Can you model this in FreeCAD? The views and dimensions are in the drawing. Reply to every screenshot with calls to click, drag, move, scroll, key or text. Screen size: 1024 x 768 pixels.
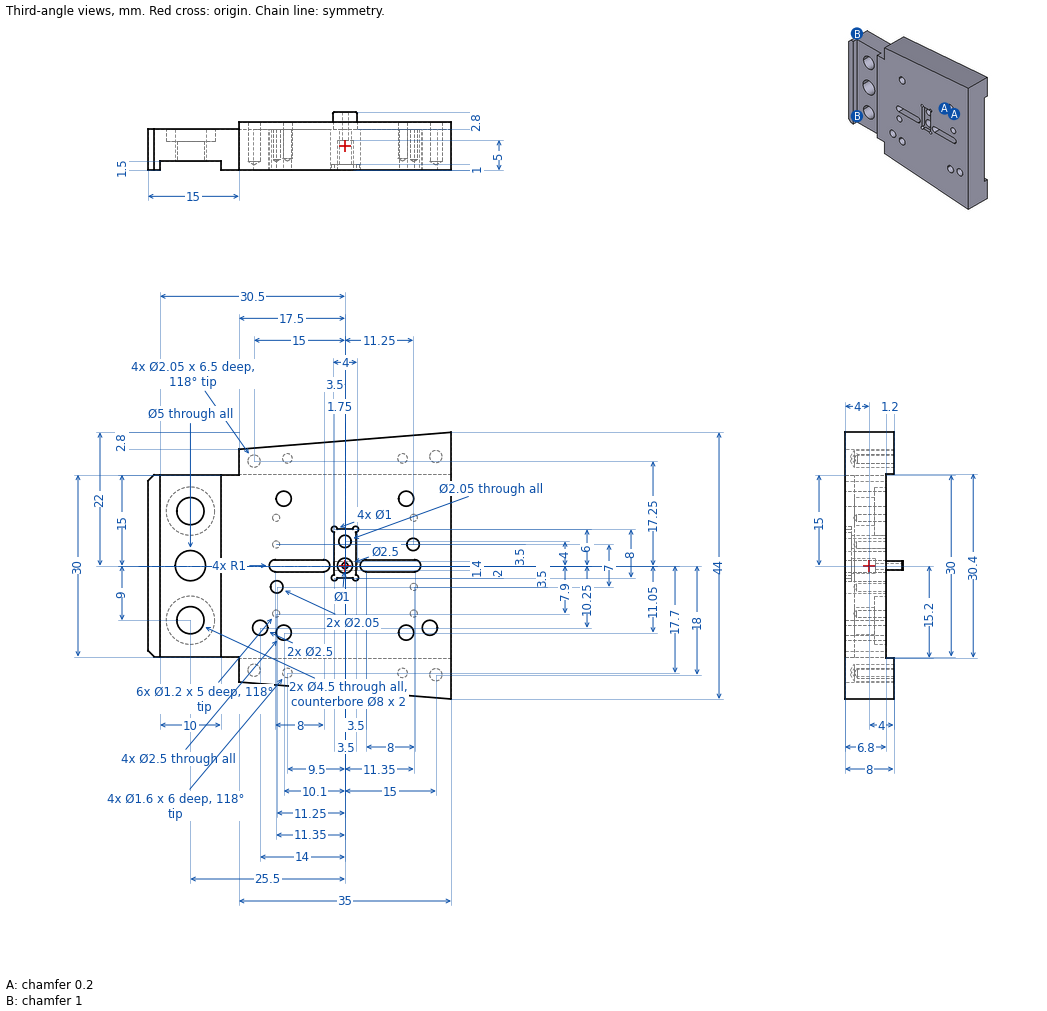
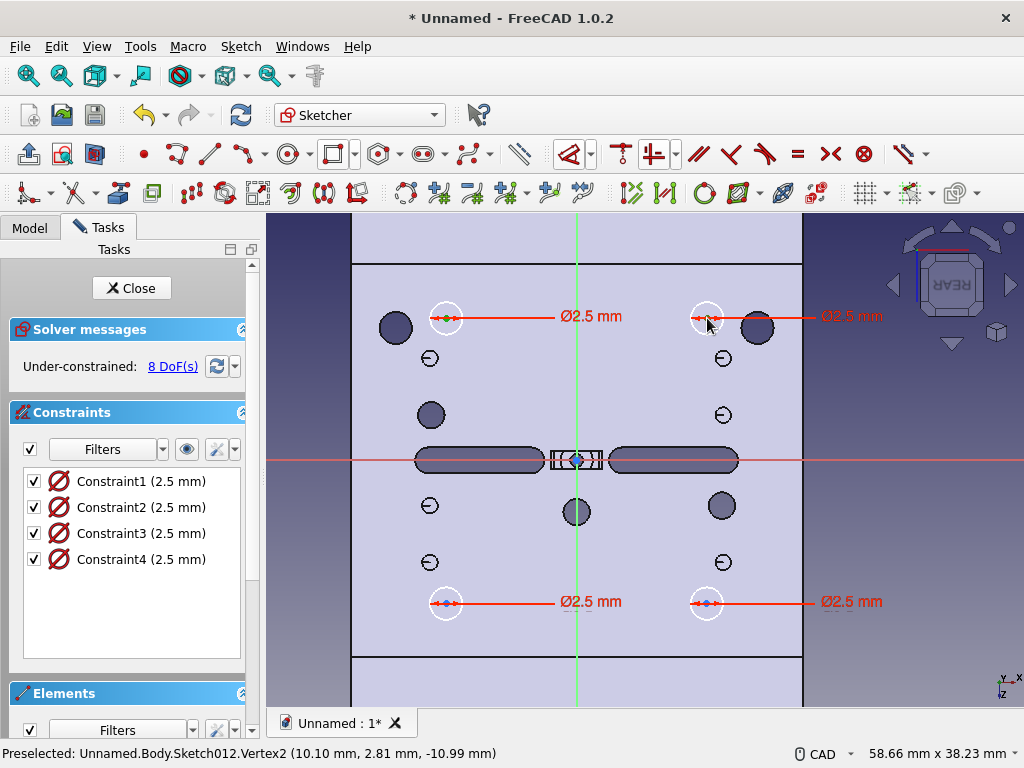
click(577, 648)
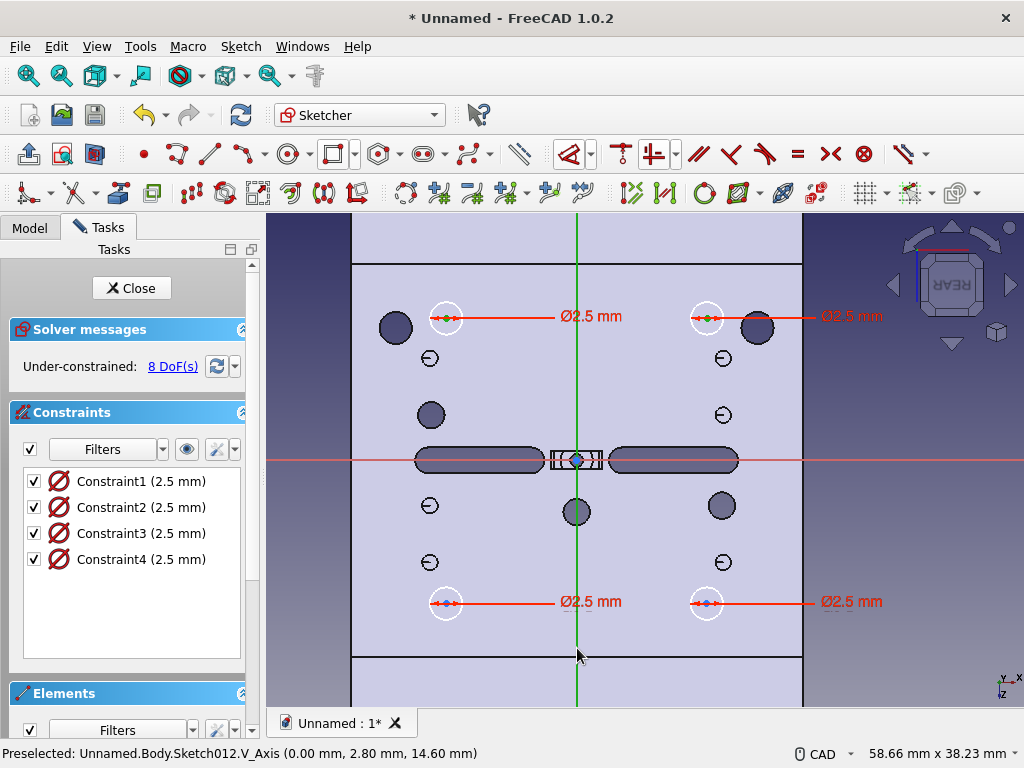
click(831, 154)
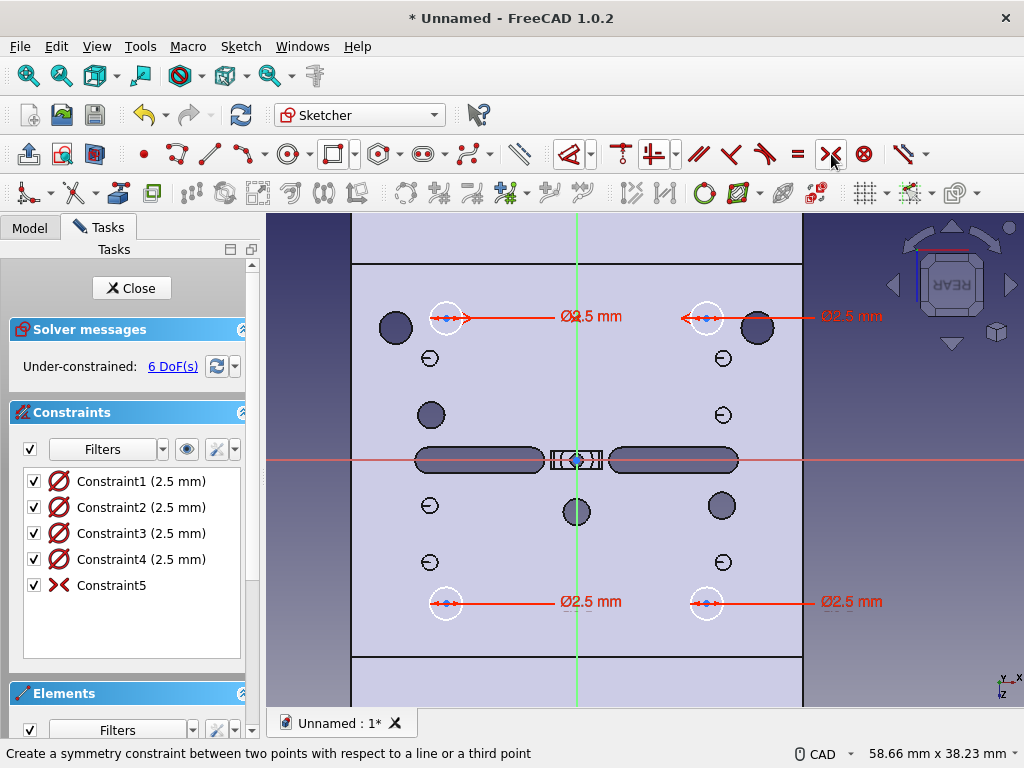
click(446, 318)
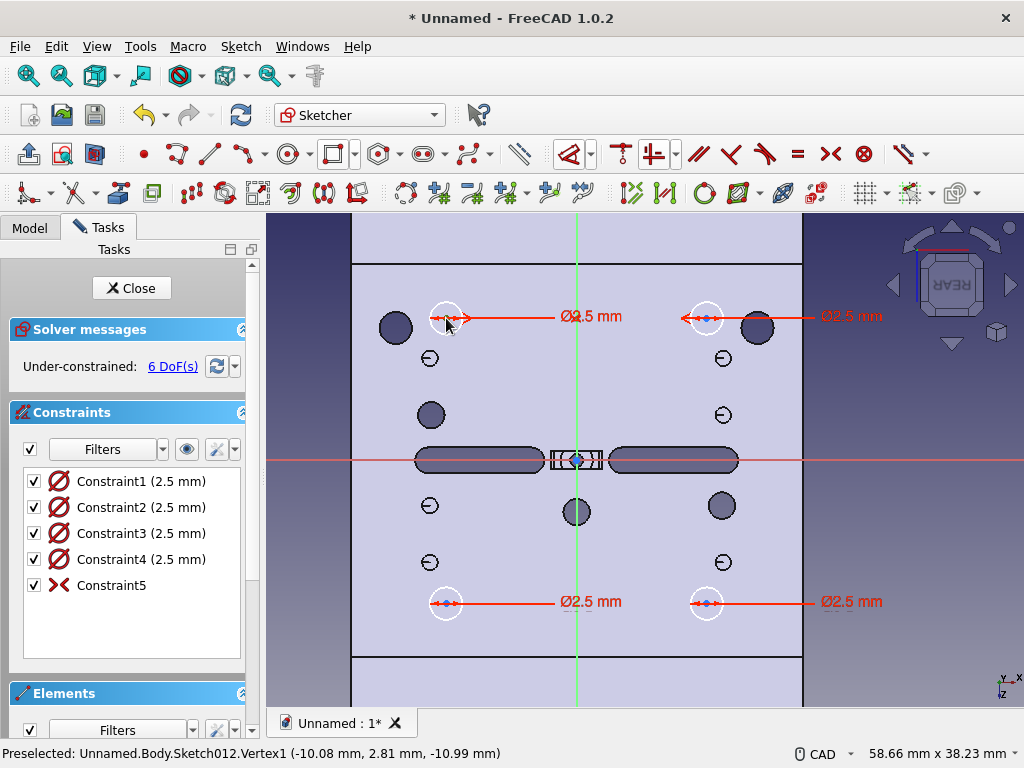
click(446, 604)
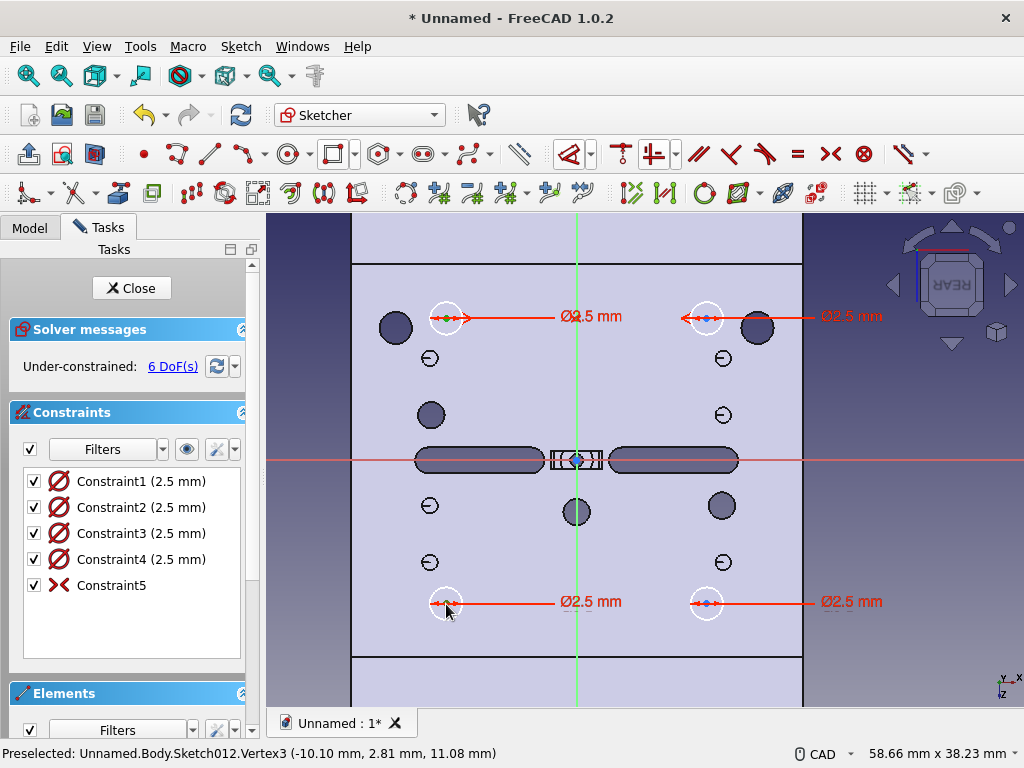
click(334, 460)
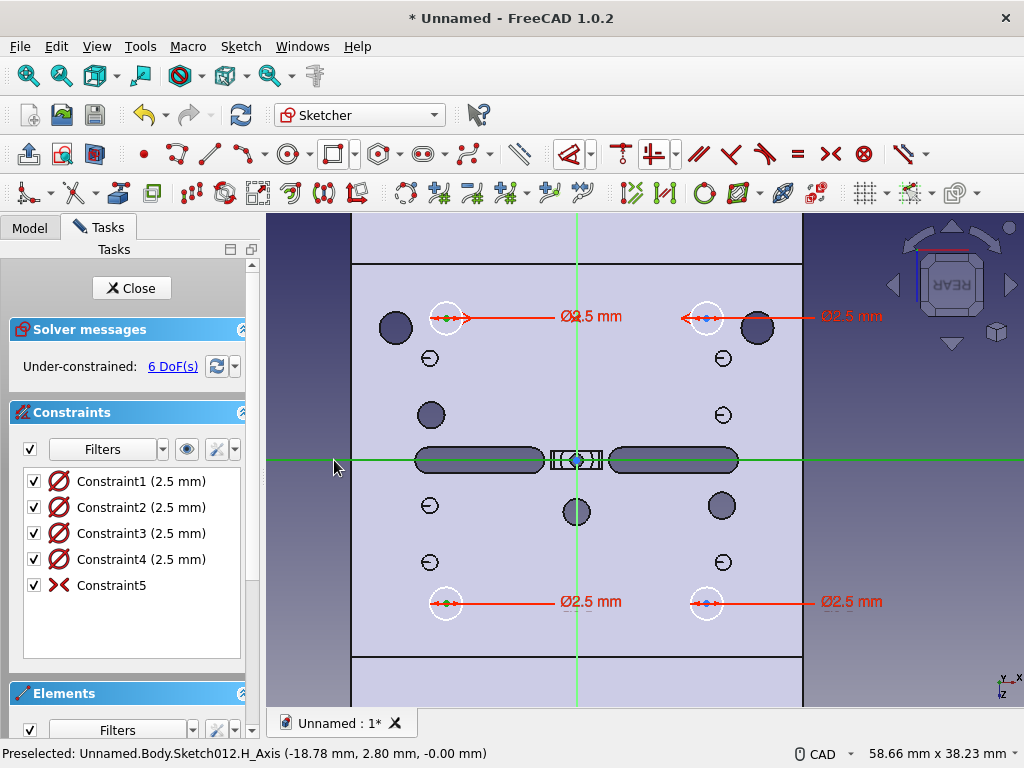
click(831, 154)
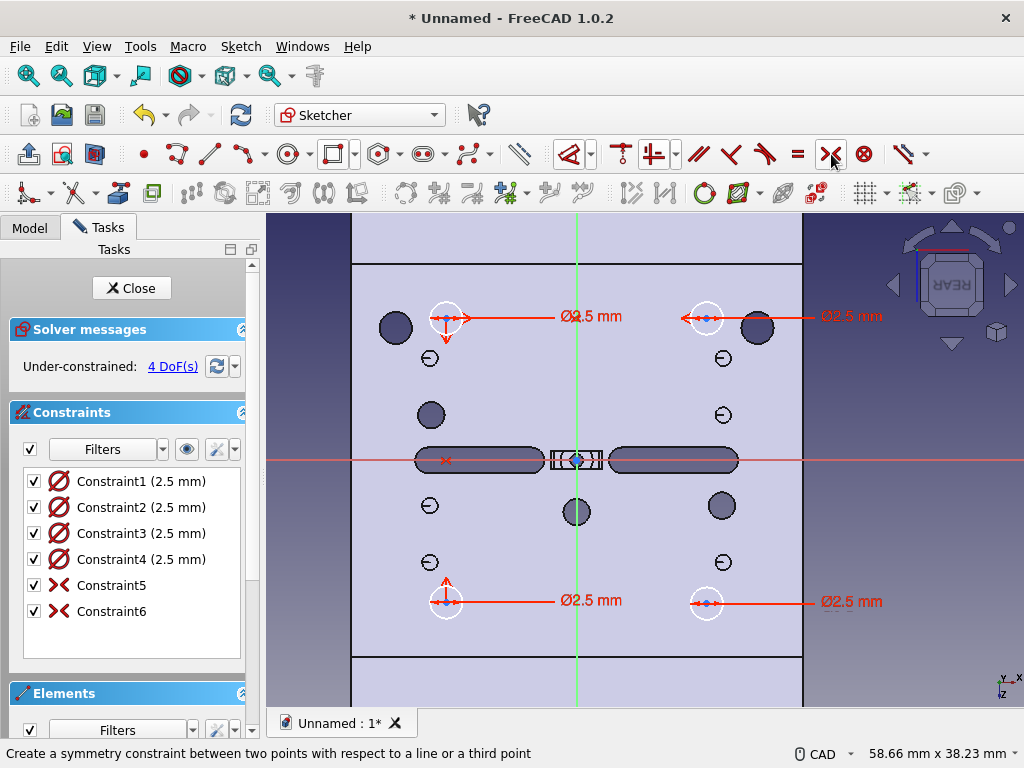
click(707, 318)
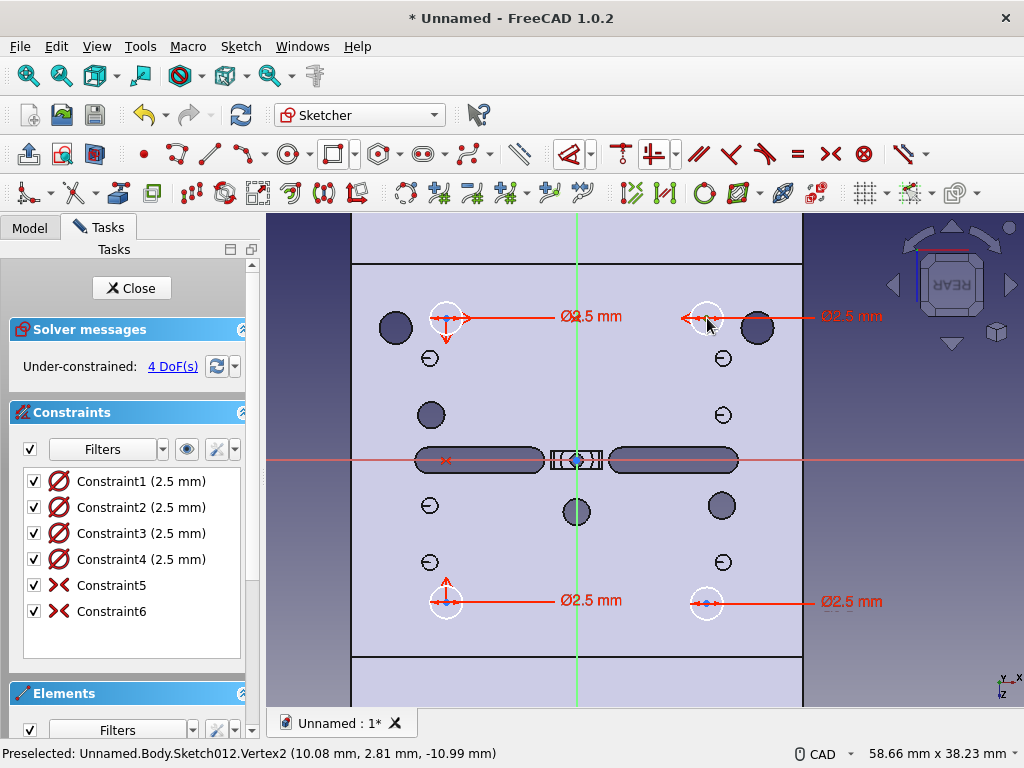
click(707, 604)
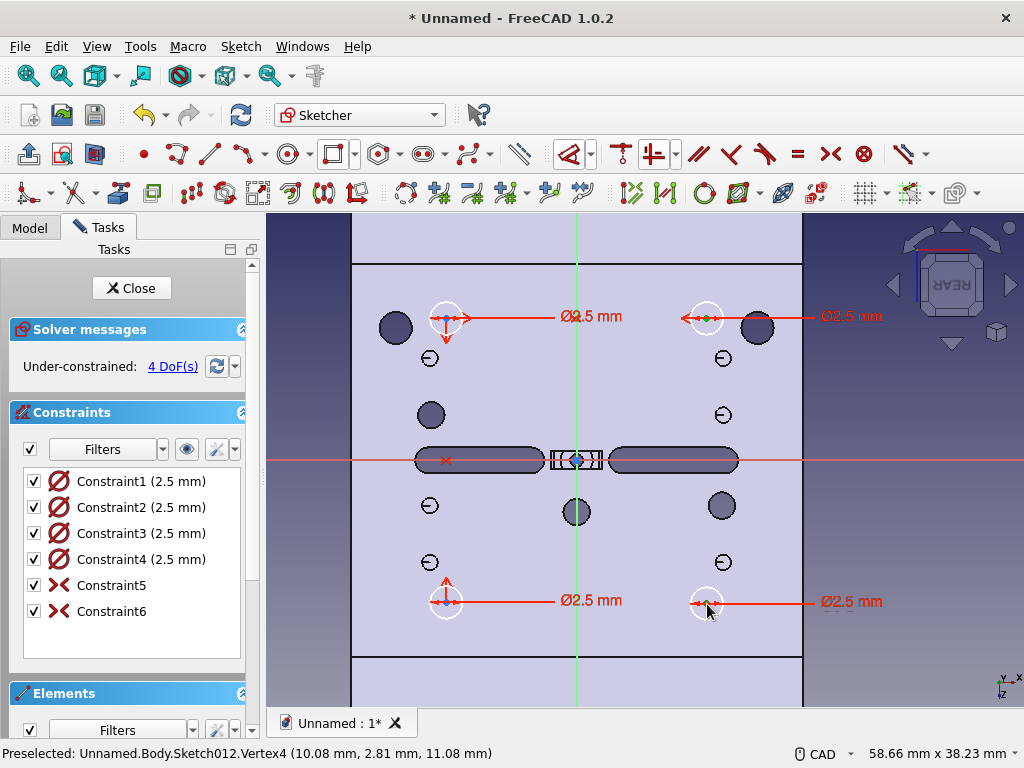
click(334, 460)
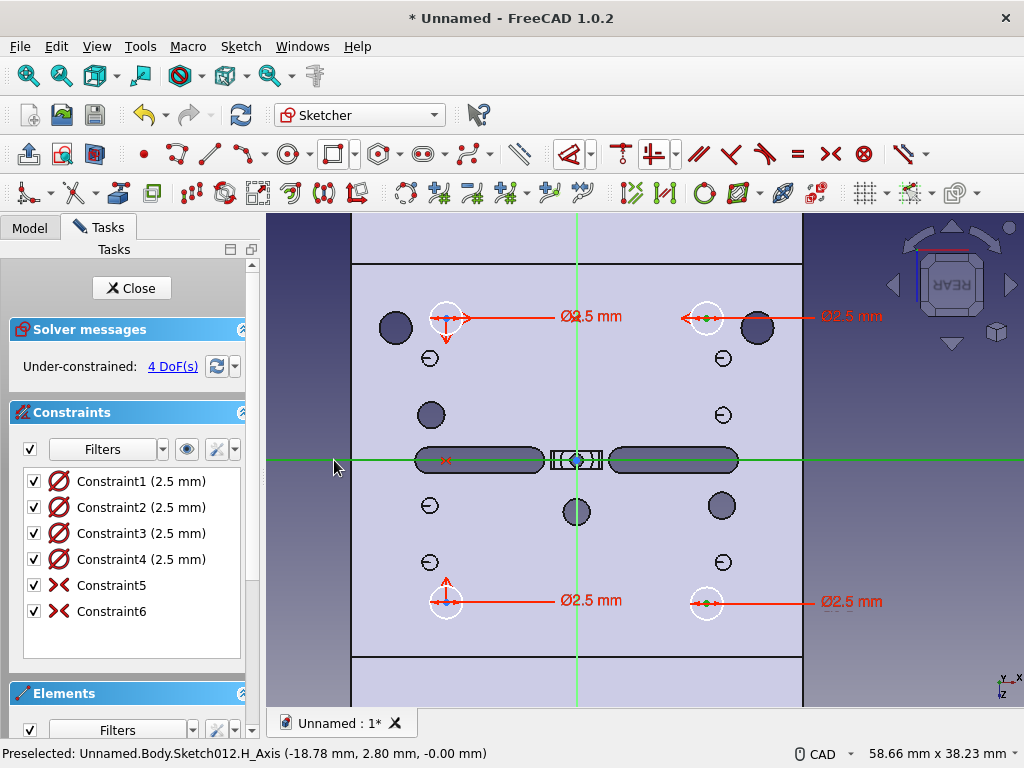
click(831, 154)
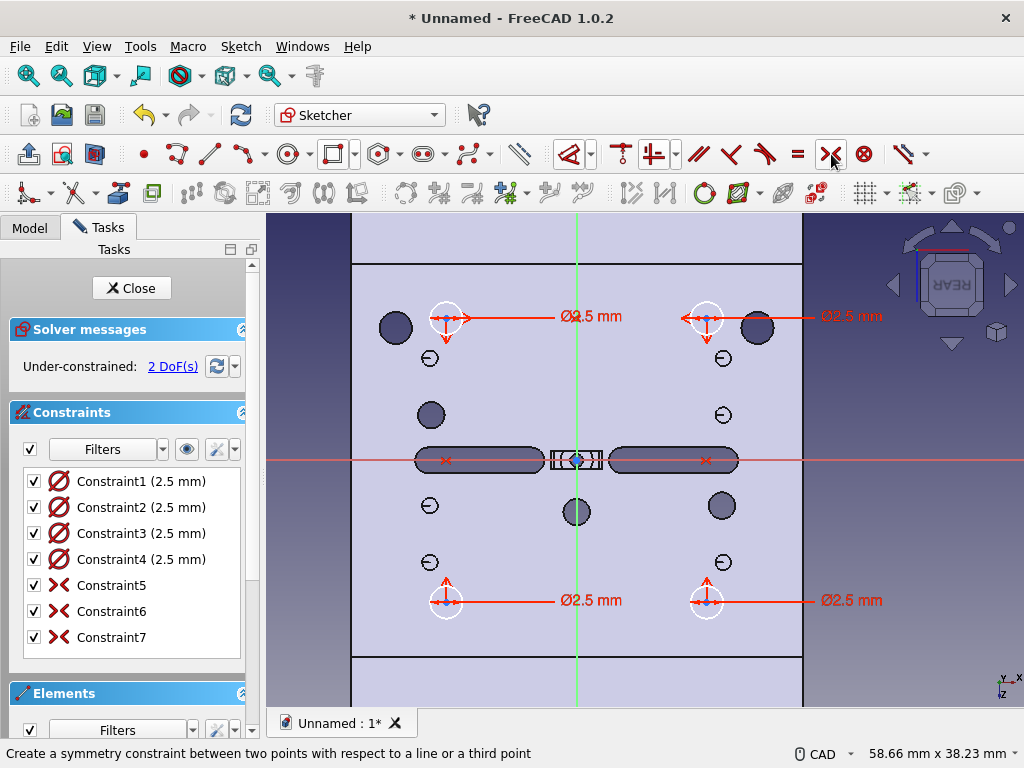
click(446, 318)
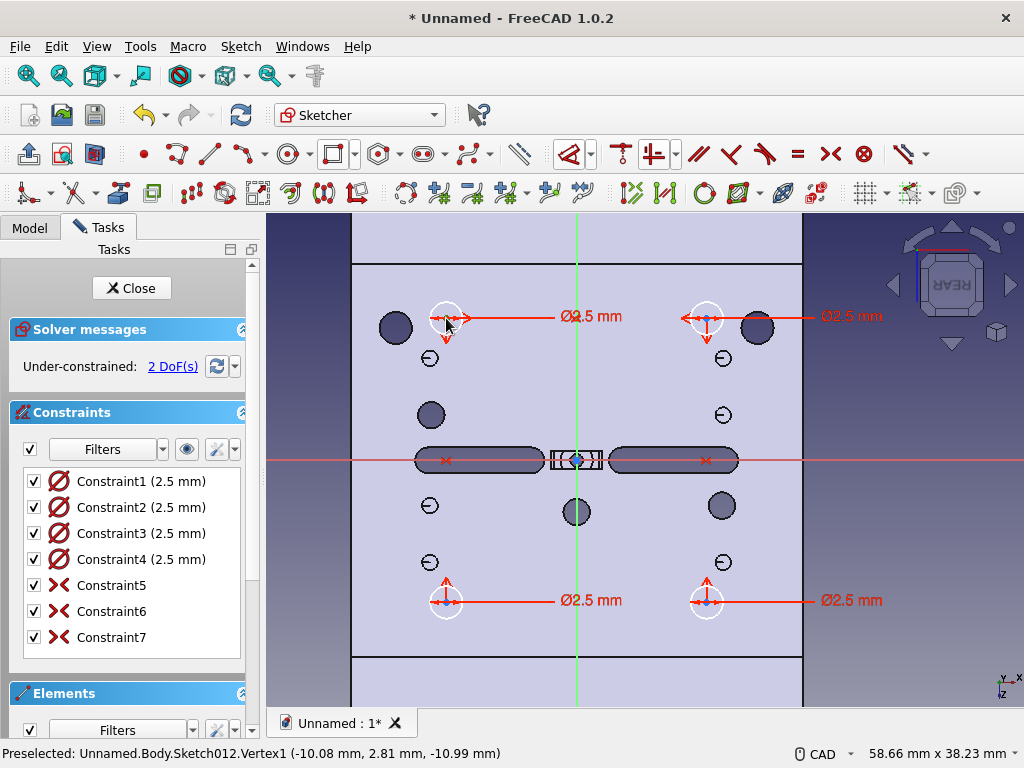
click(590, 154)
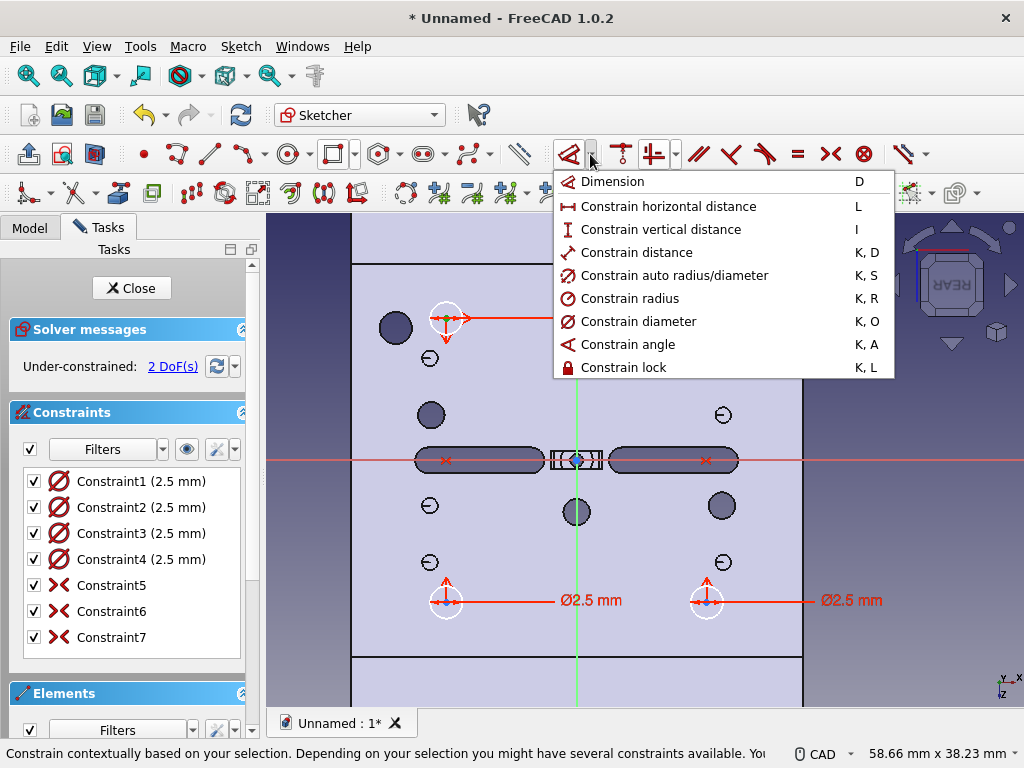
click(724, 206)